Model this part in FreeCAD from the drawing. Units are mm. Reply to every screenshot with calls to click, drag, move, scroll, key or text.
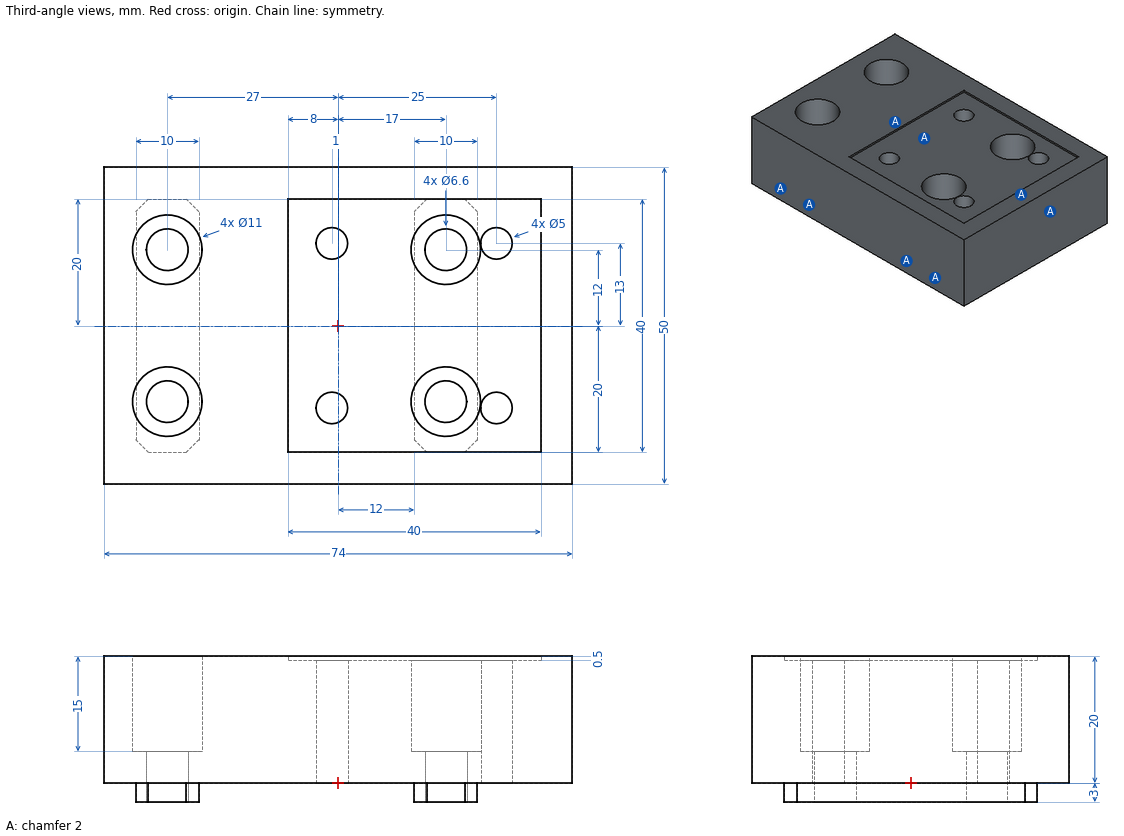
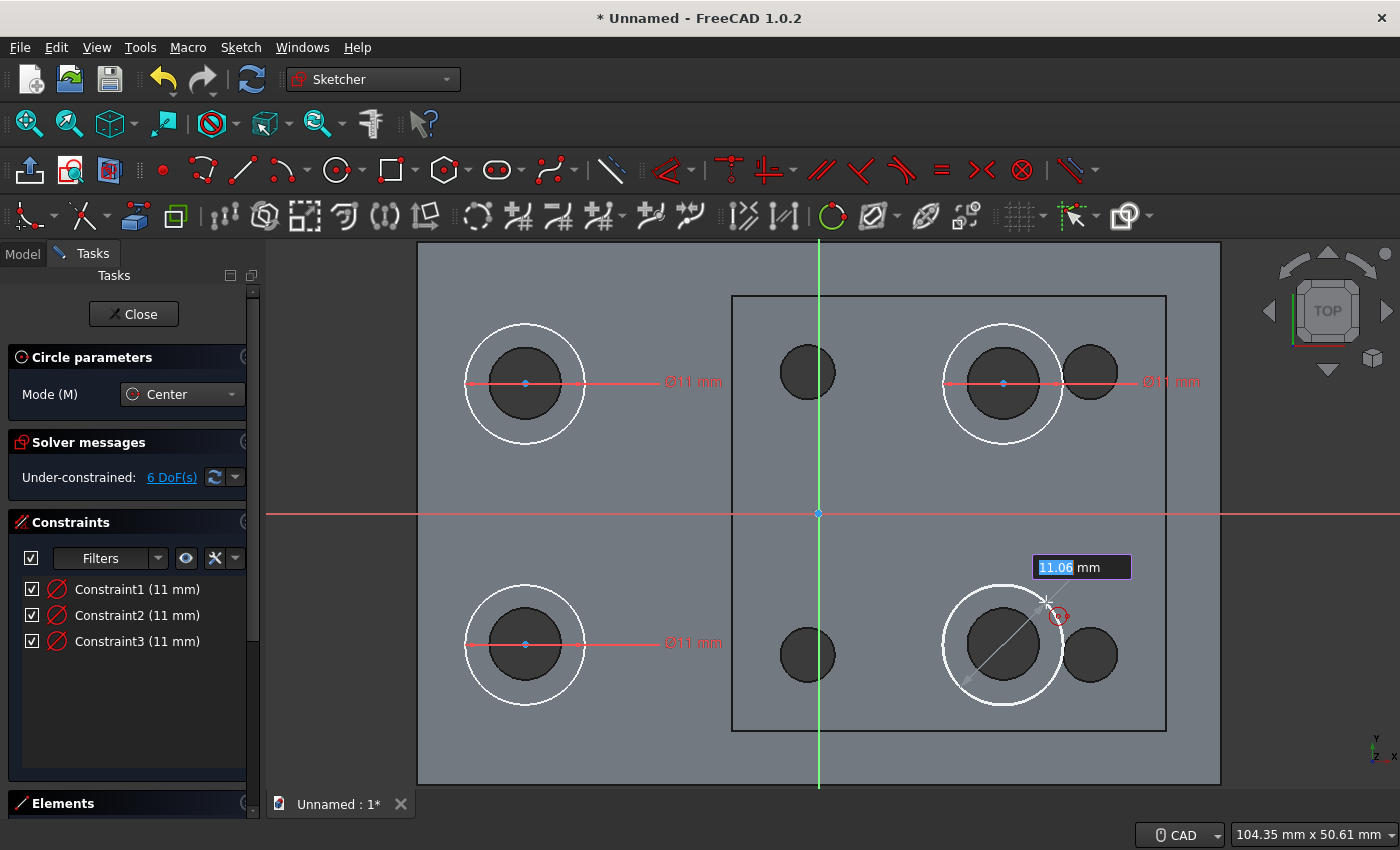
text(11)
key(Return)
key(Escape)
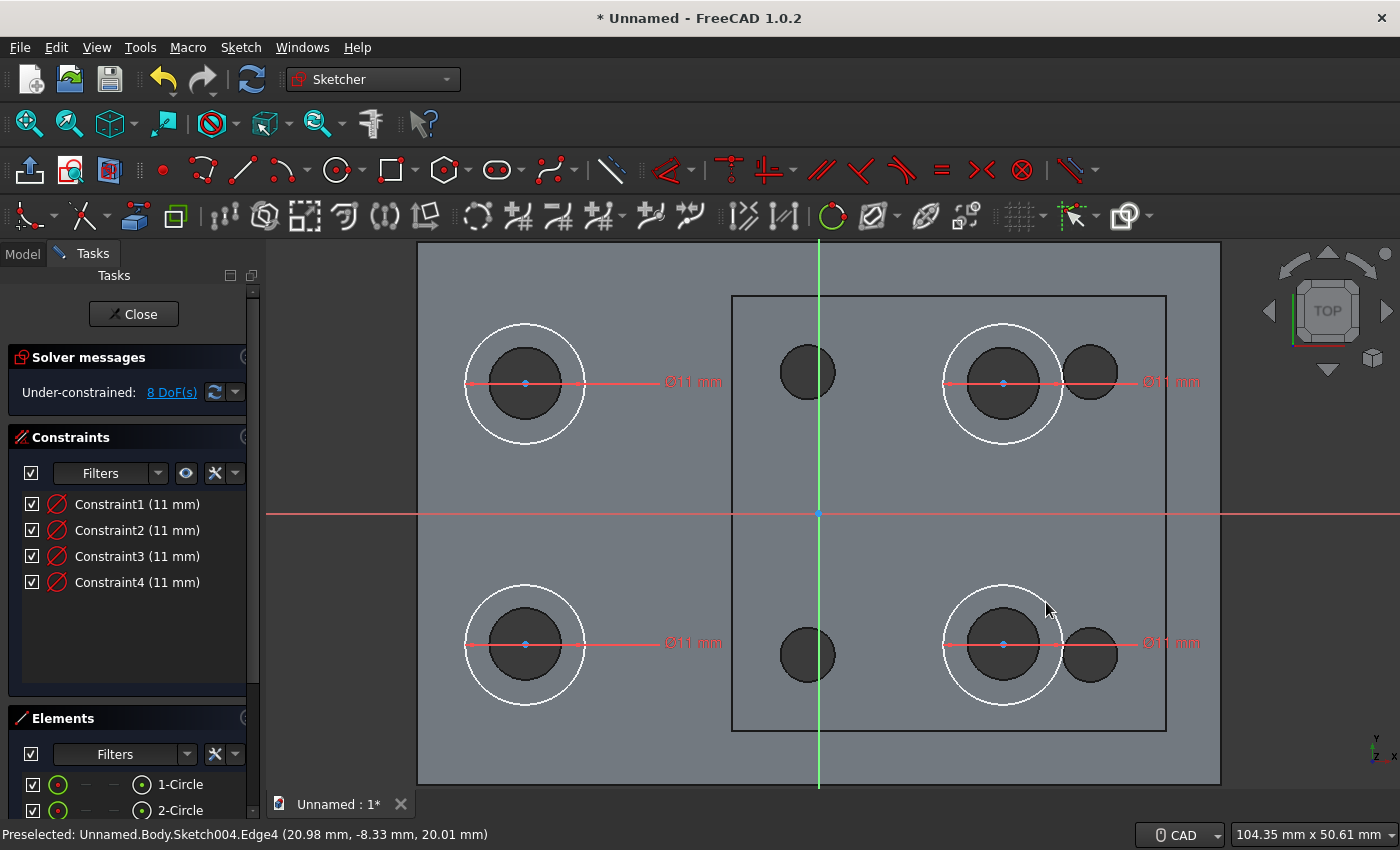
click(525, 384)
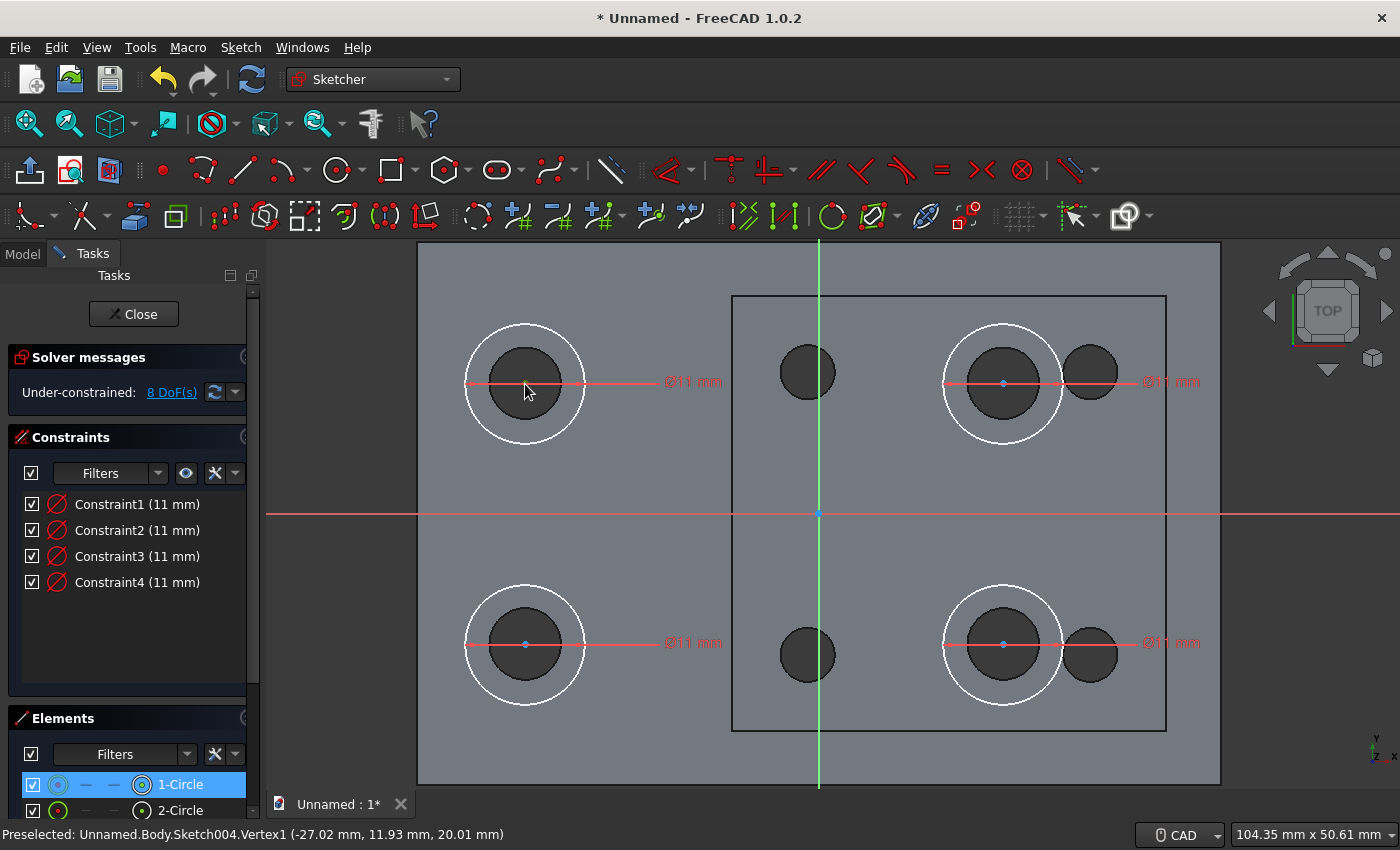
click(525, 645)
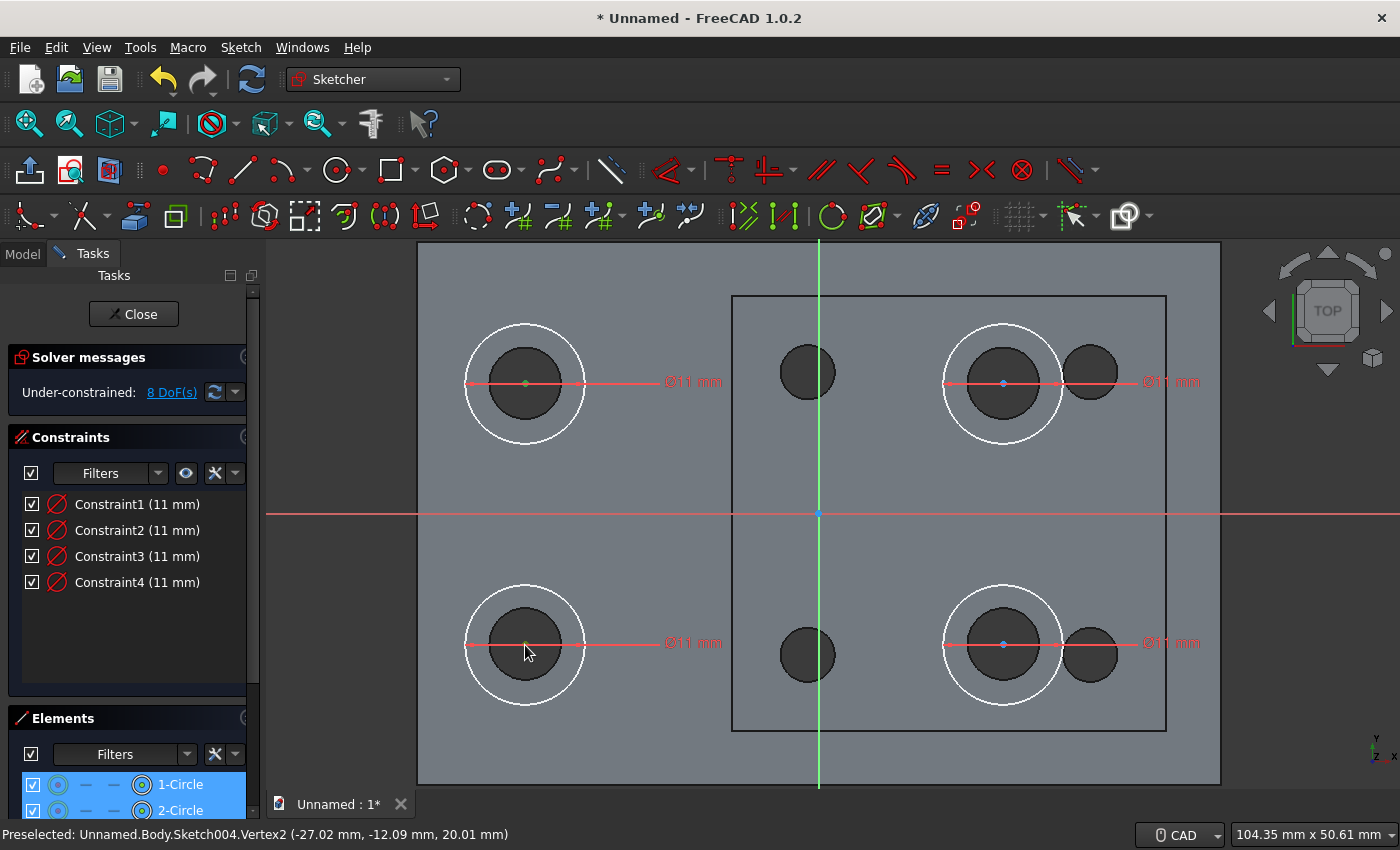
click(361, 514)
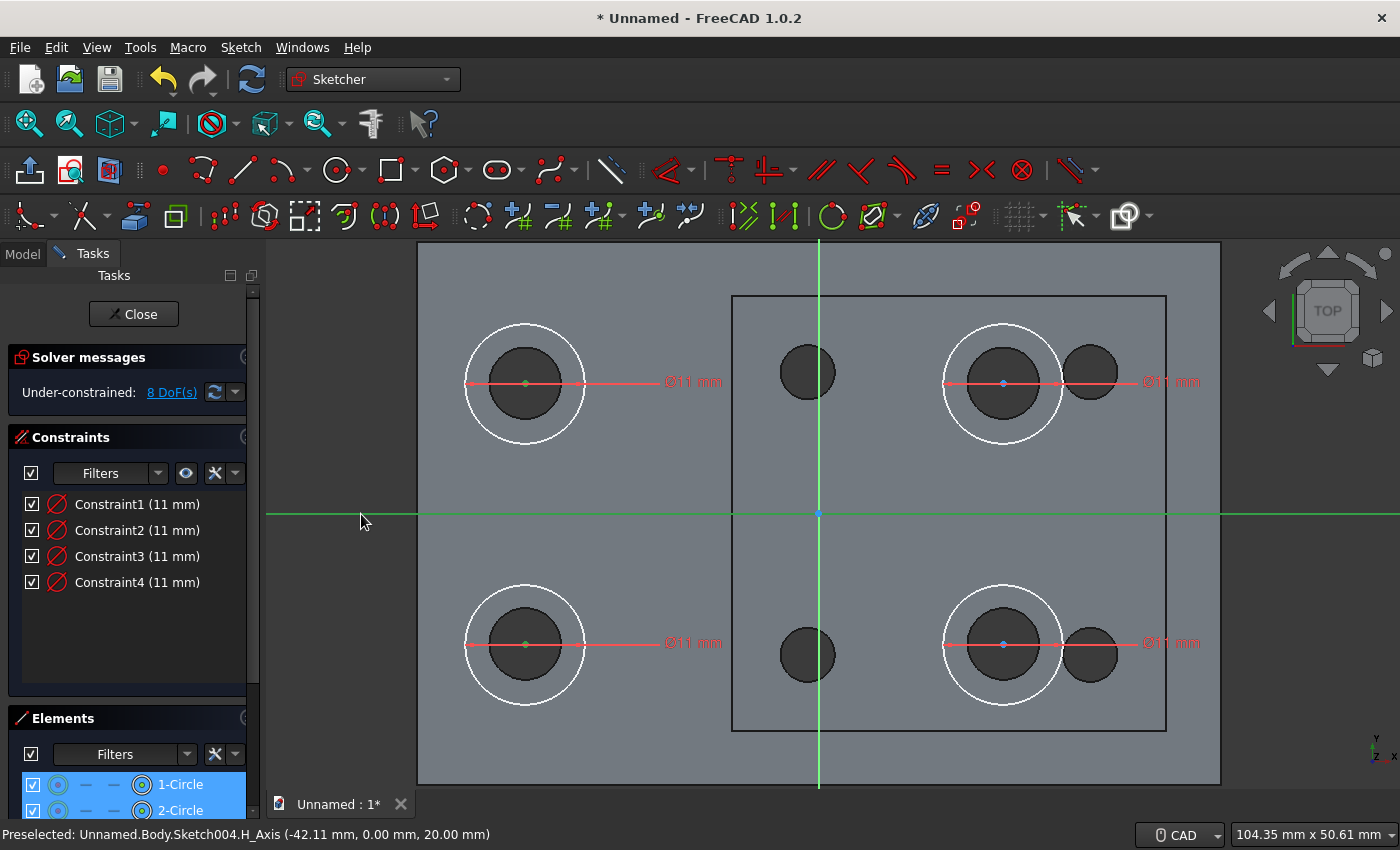
click(982, 170)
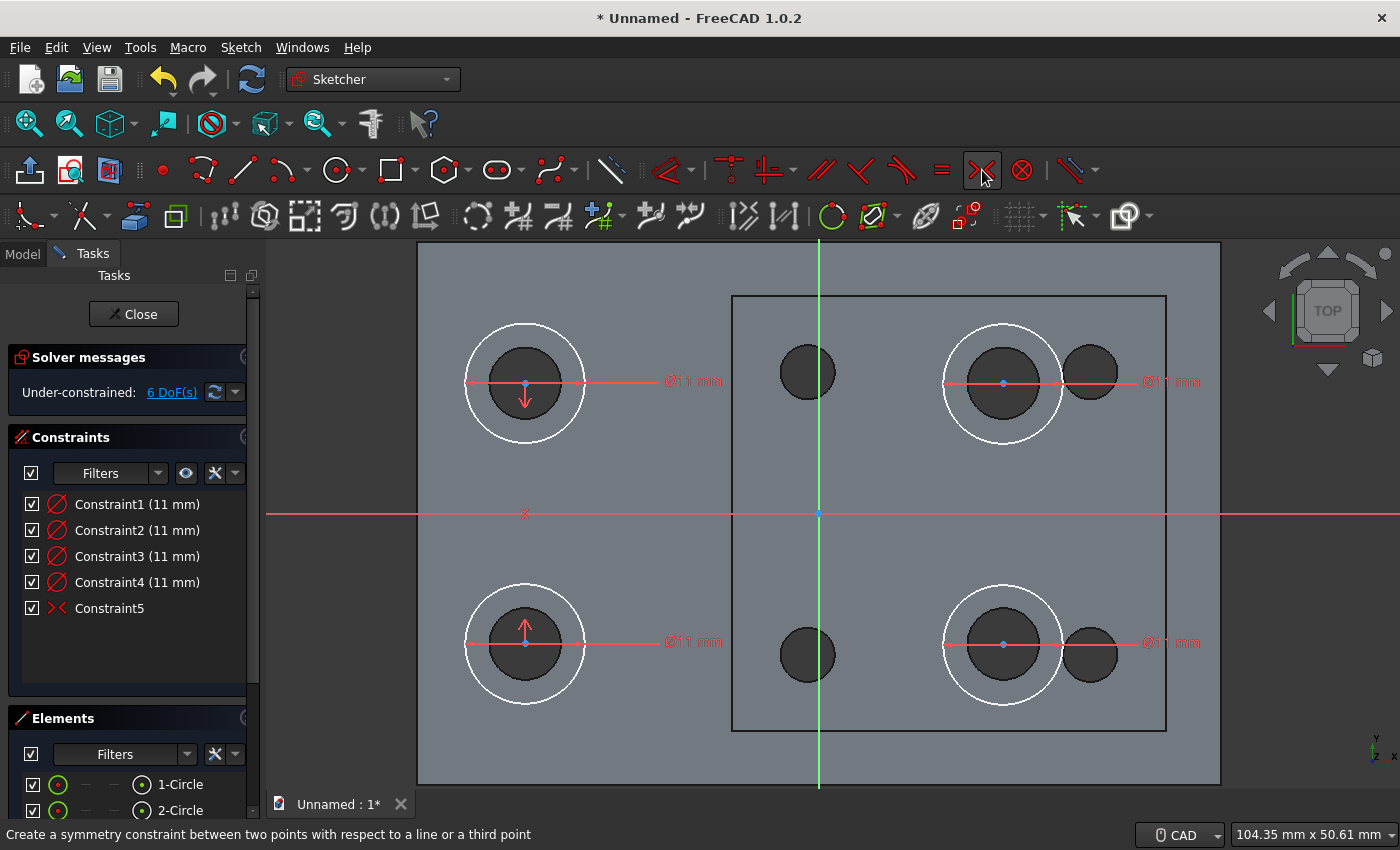
click(1003, 384)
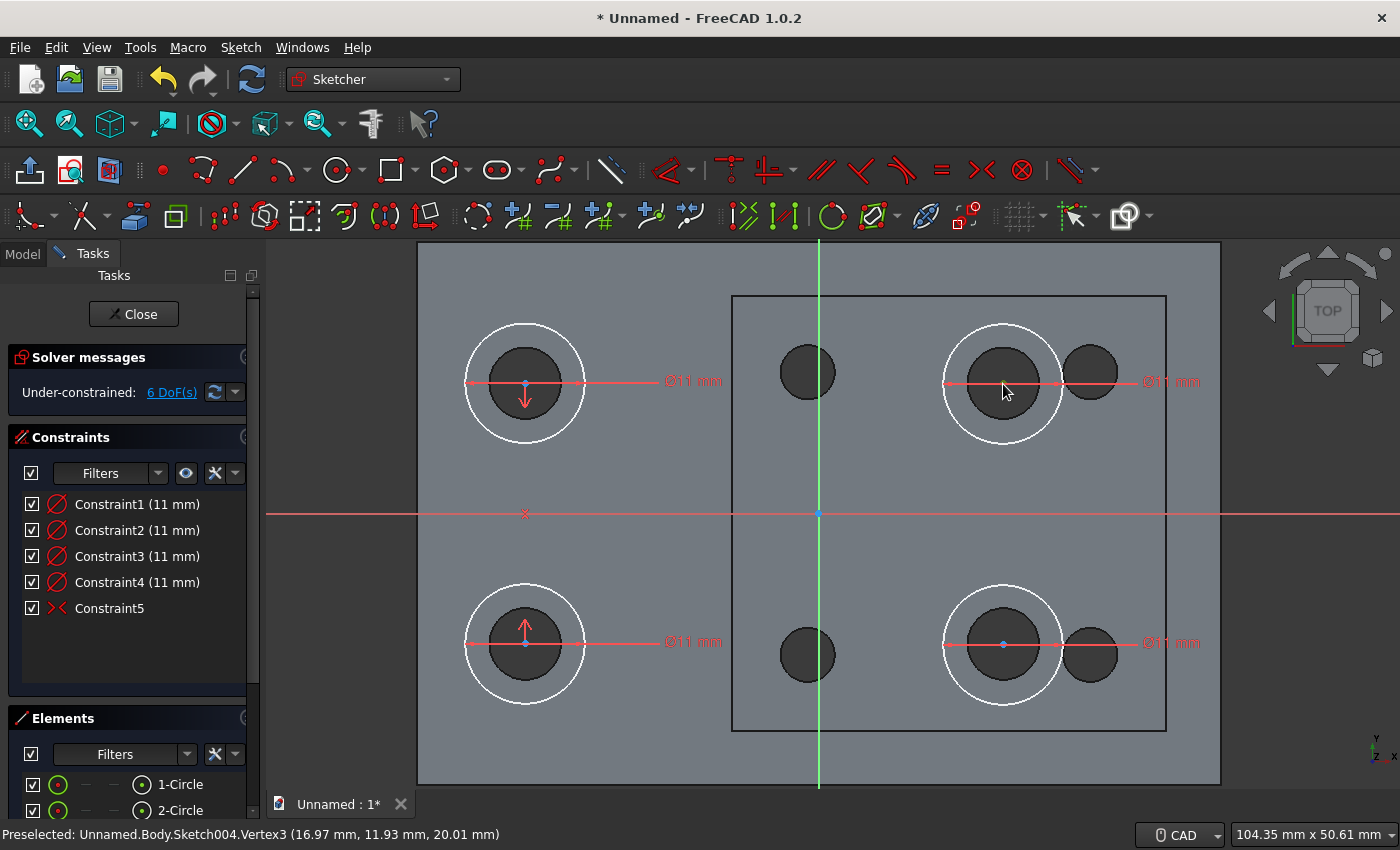
click(1003, 645)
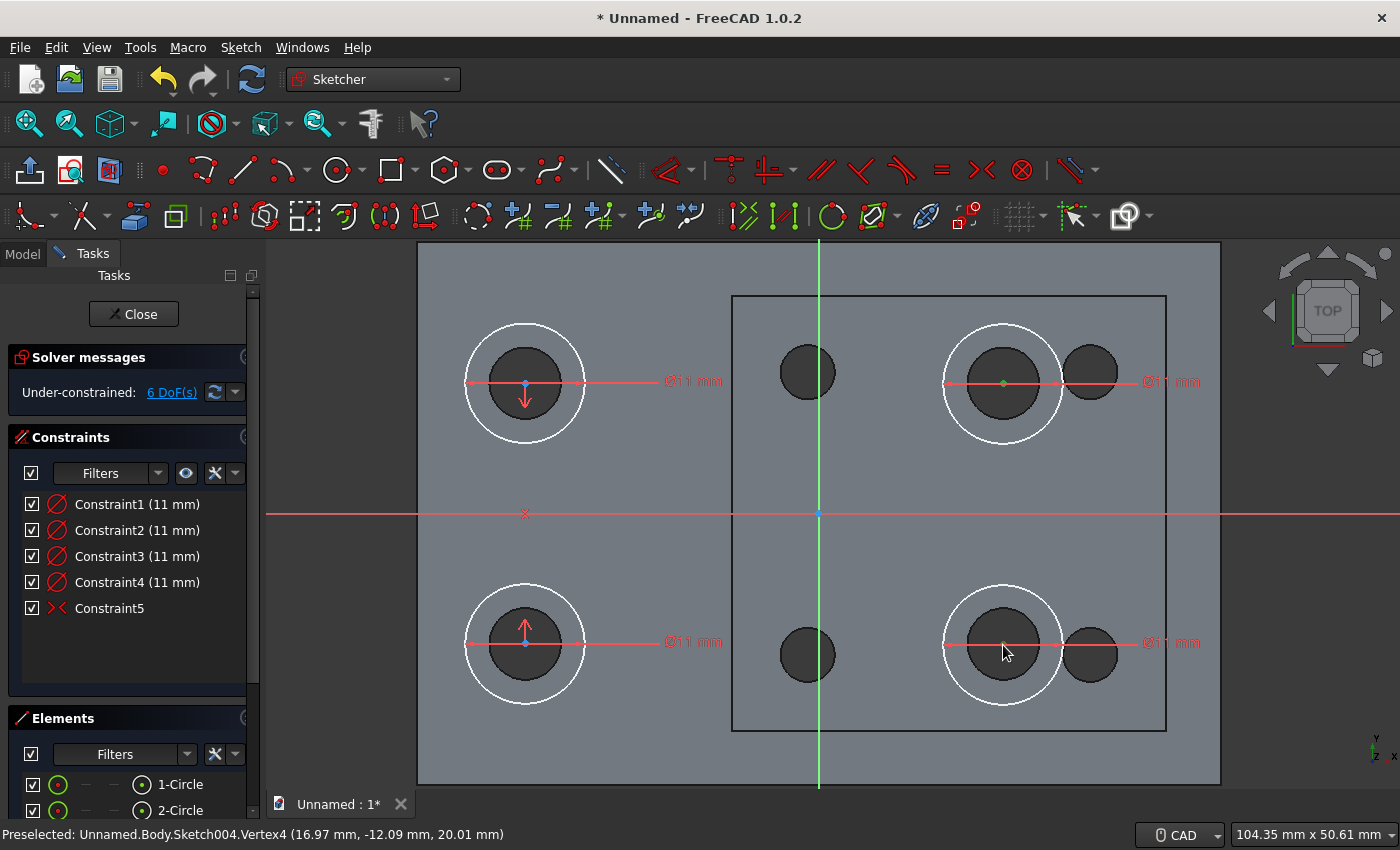
click(361, 514)